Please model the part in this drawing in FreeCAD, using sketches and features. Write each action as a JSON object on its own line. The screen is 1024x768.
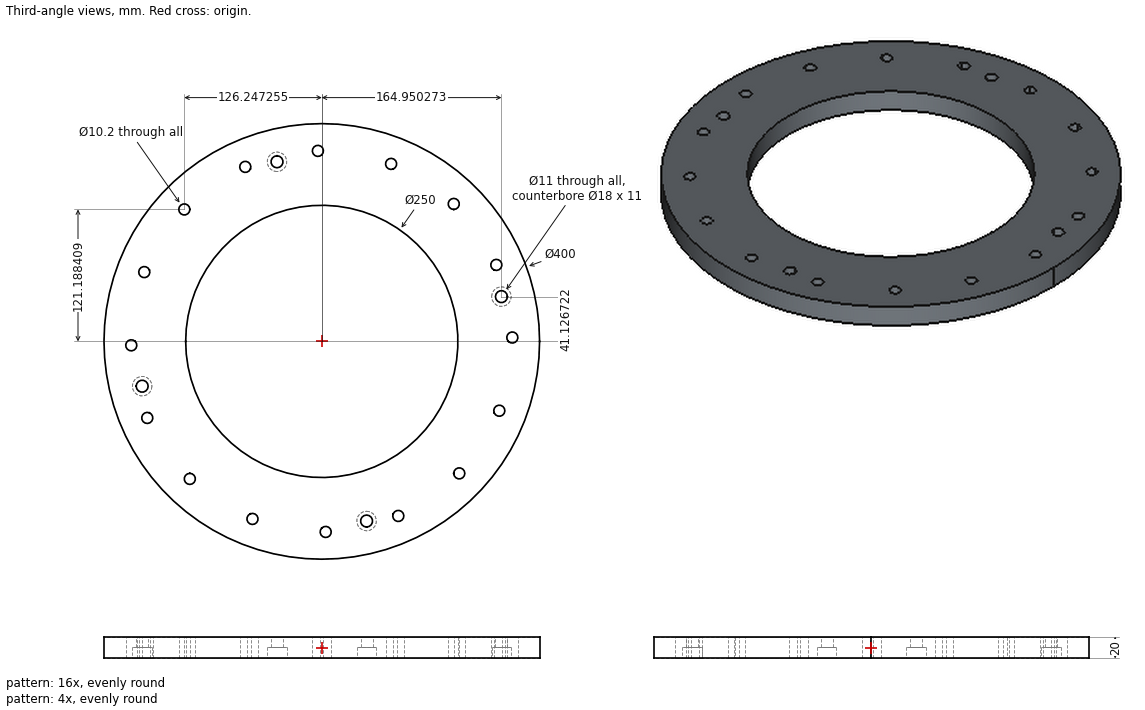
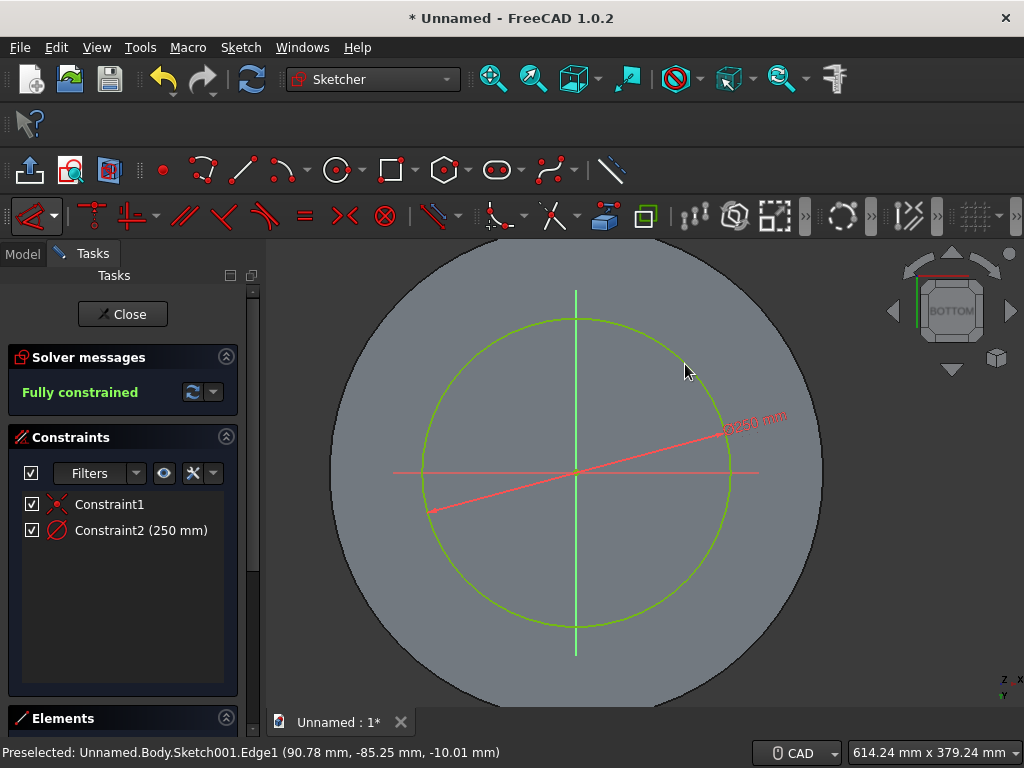
{"action": "left_click", "coordinate": [123, 314]}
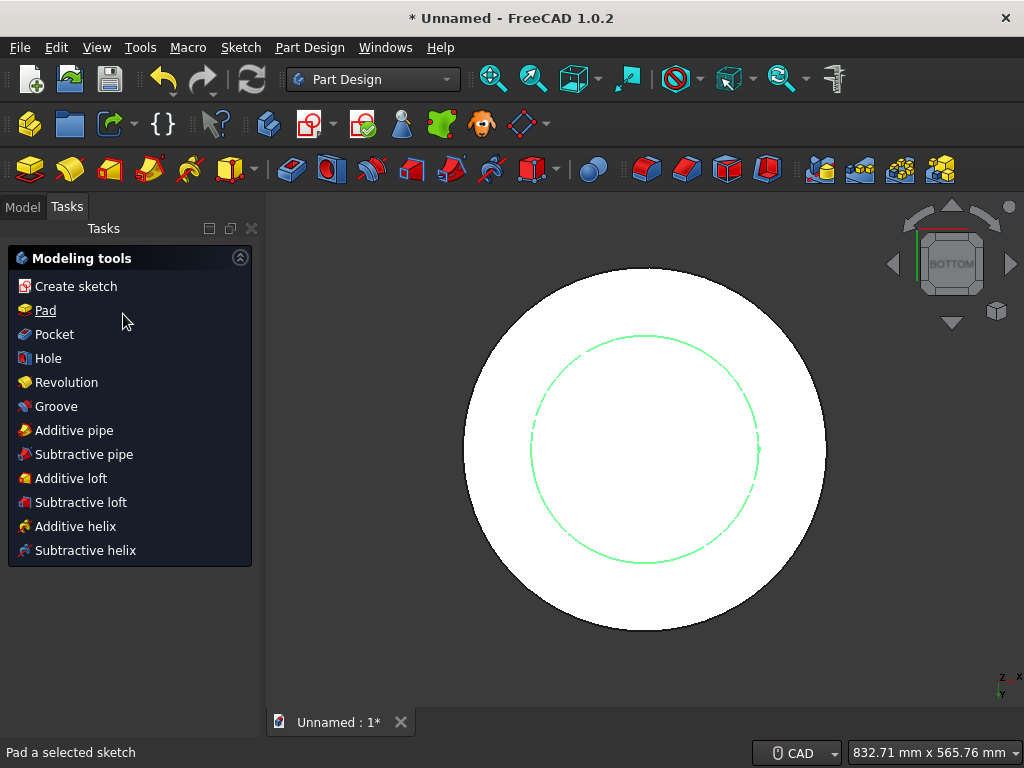
{"action": "left_click", "coordinate": [292, 170]}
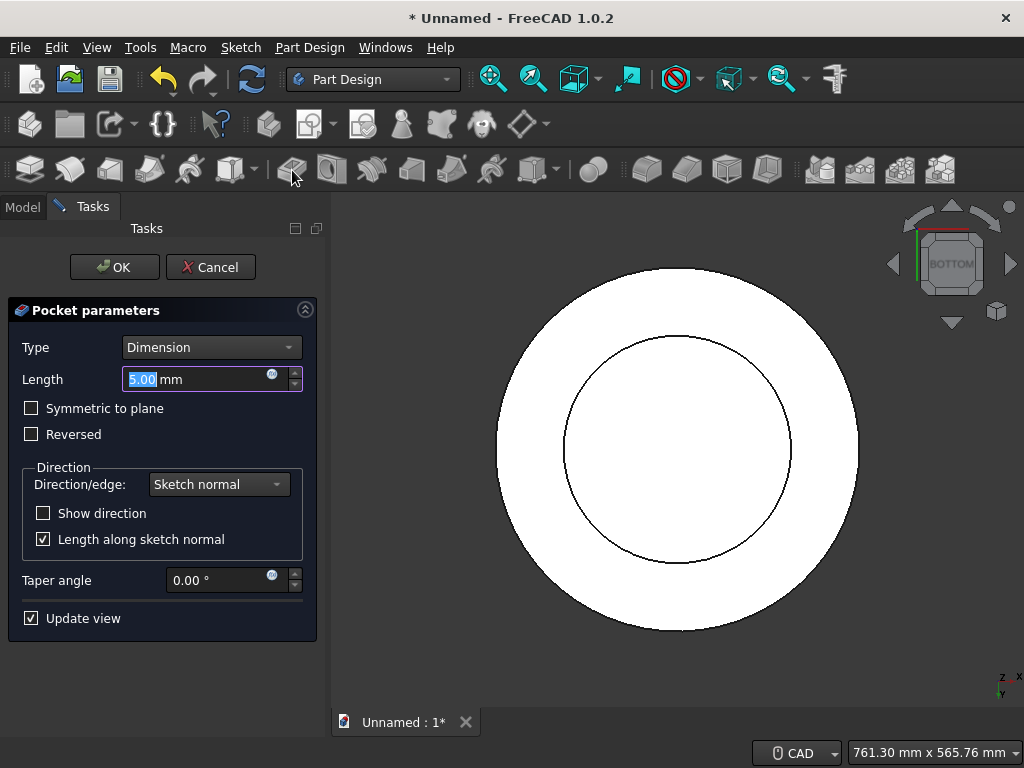
{"action": "left_click", "coordinate": [212, 348]}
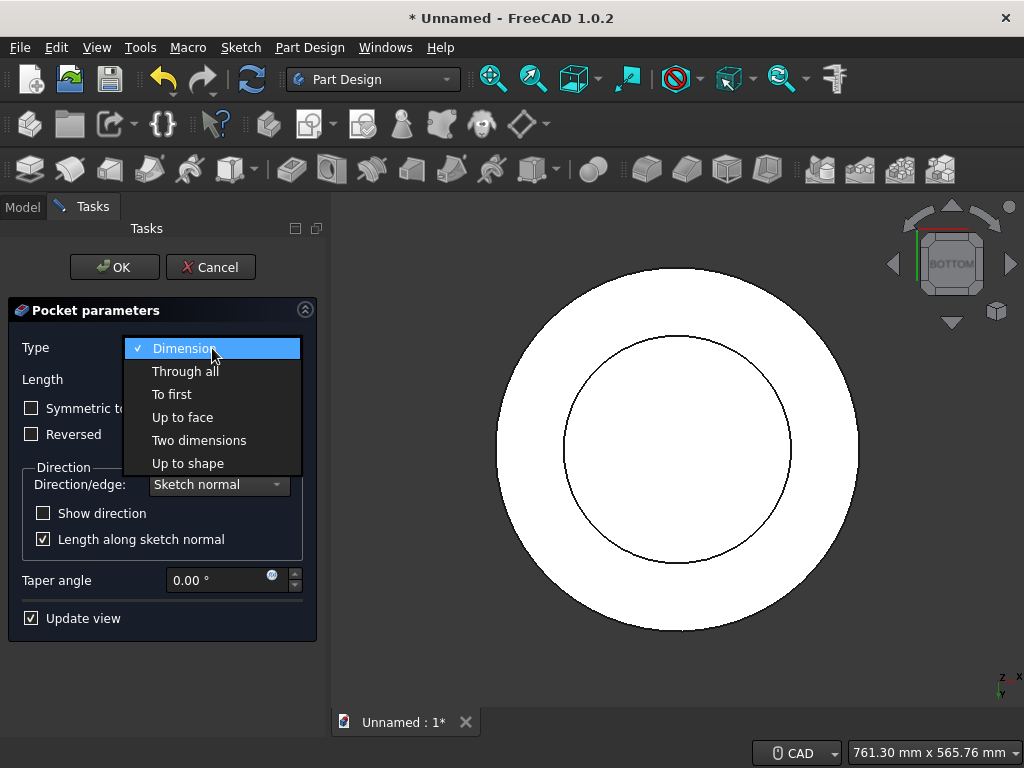
{"action": "left_click", "coordinate": [212, 372]}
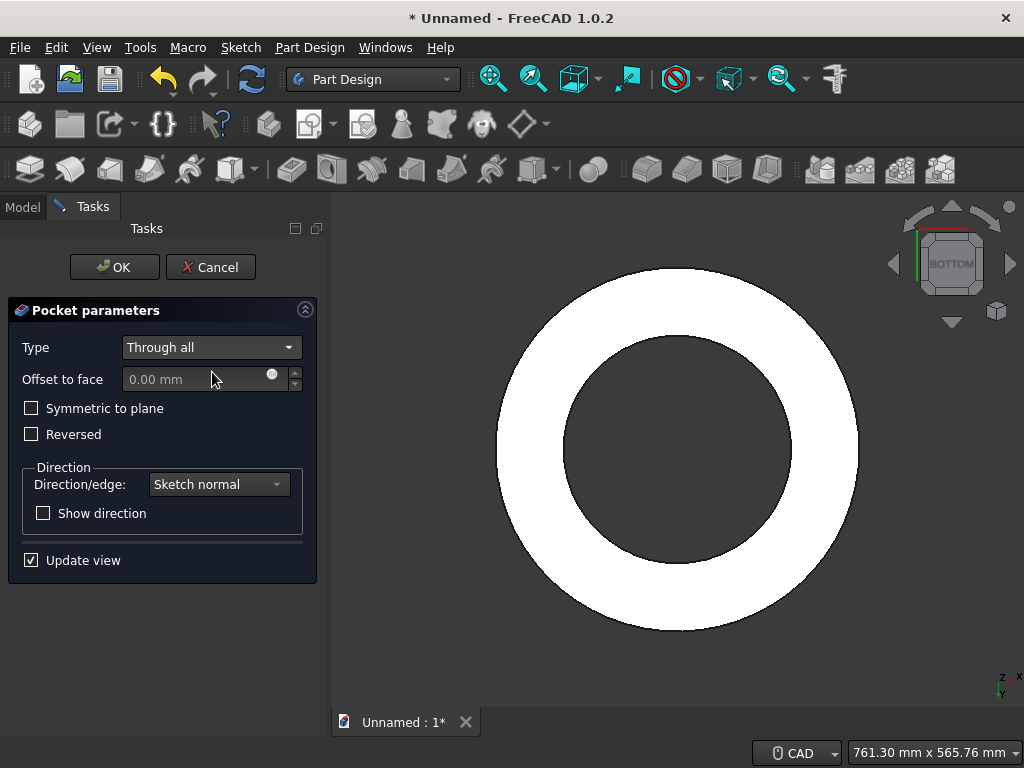
{"action": "left_click", "coordinate": [115, 267]}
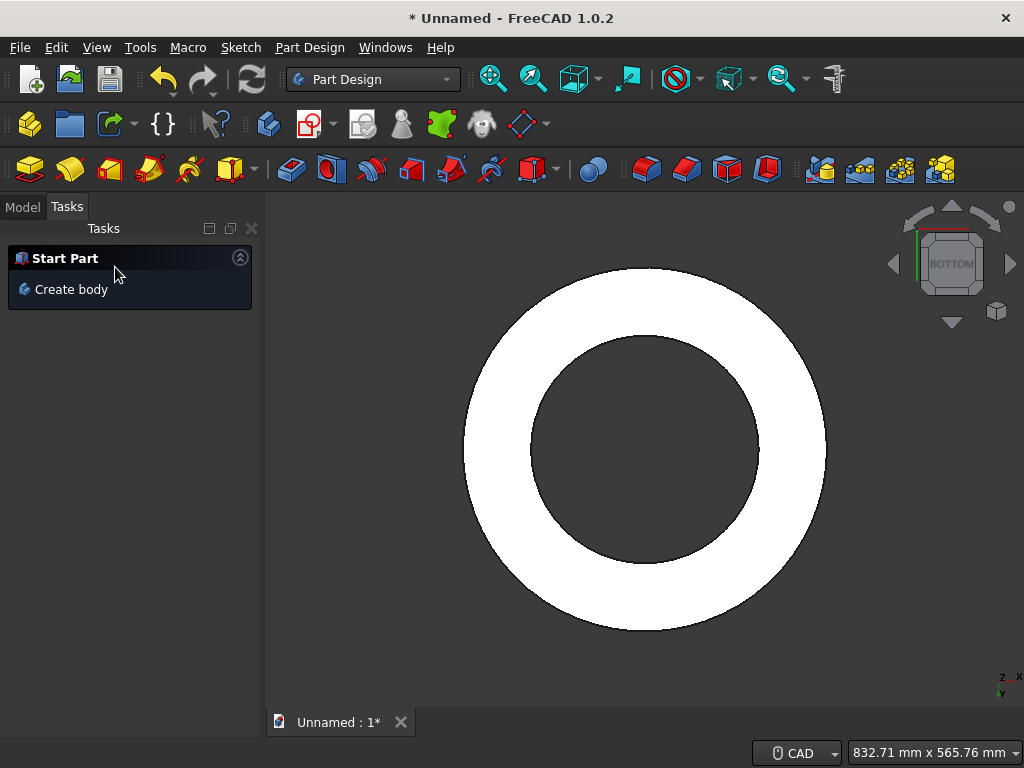
{"action": "left_click", "coordinate": [749, 553]}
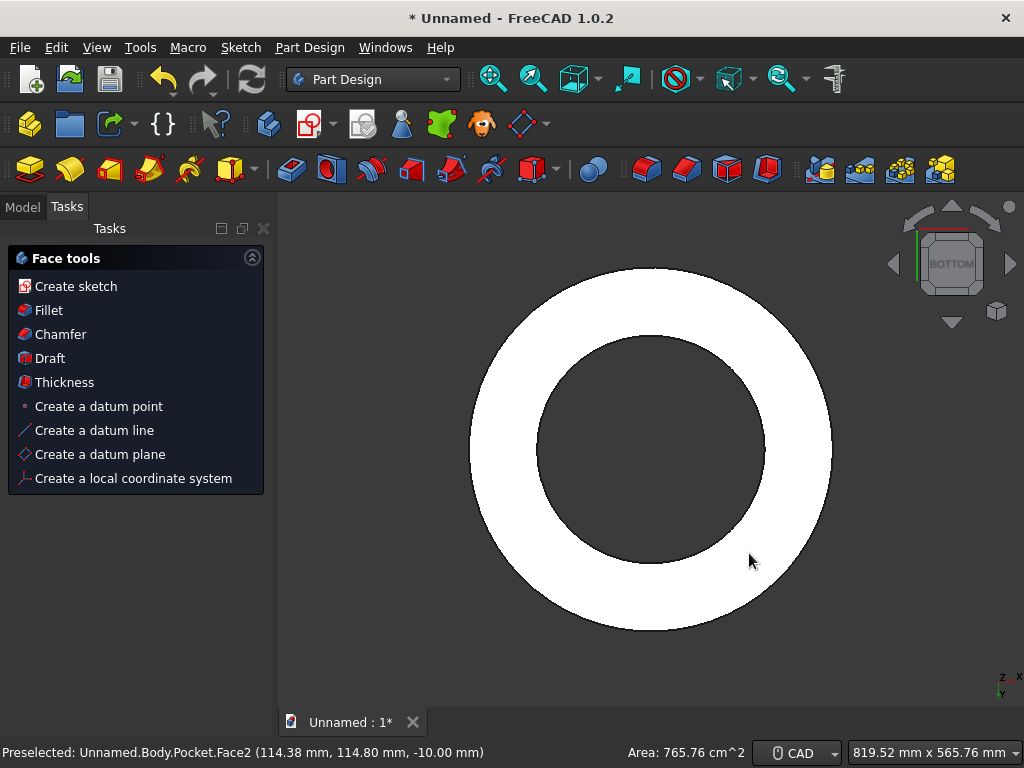
{"action": "left_click", "coordinate": [310, 124]}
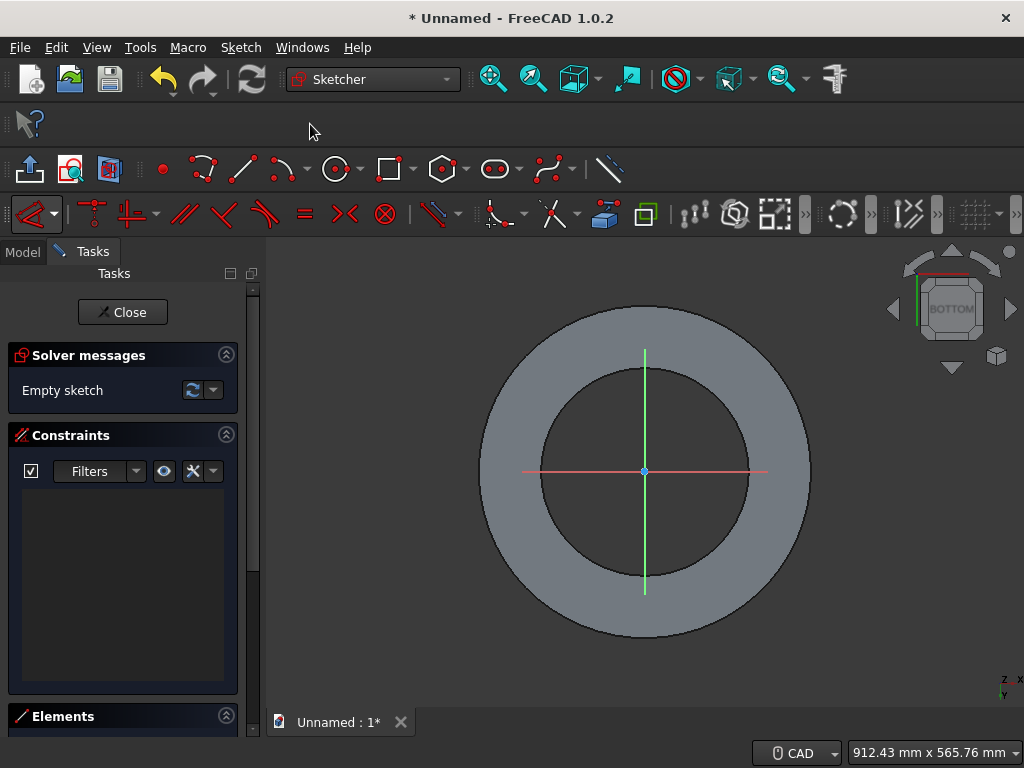
{"action": "scroll", "coordinate": [538, 578], "scroll_direction": "up", "scroll_amount": 15}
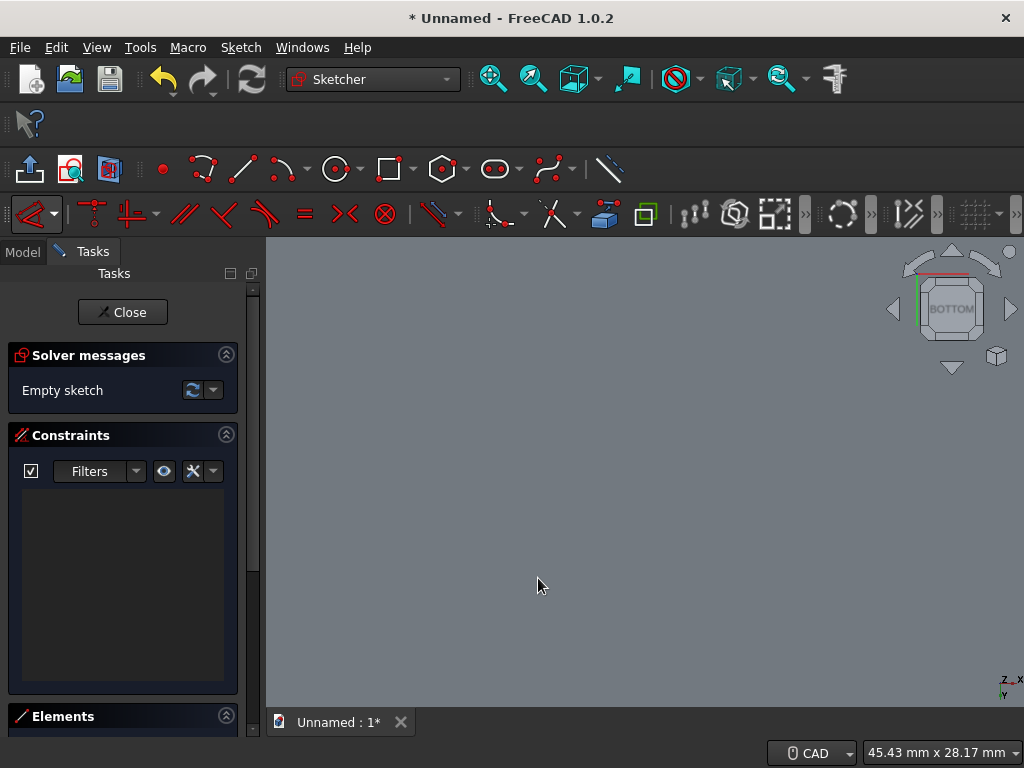
{"action": "scroll", "coordinate": [565, 439], "scroll_direction": "up", "scroll_amount": 3}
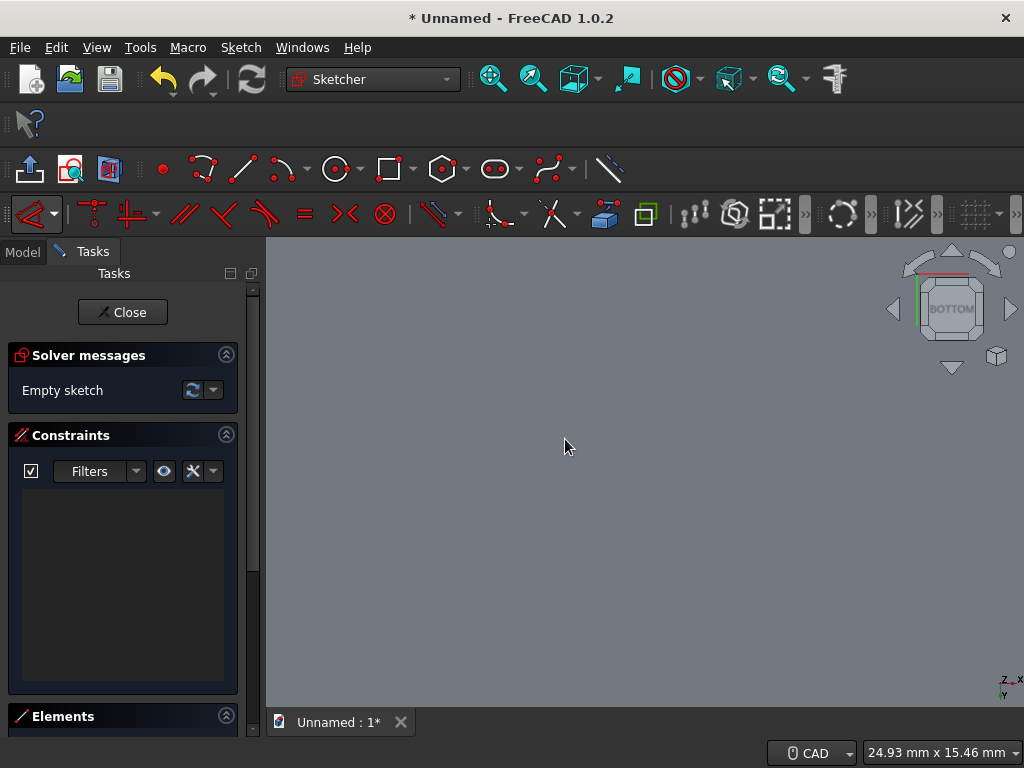
{"action": "left_click", "coordinate": [336, 170]}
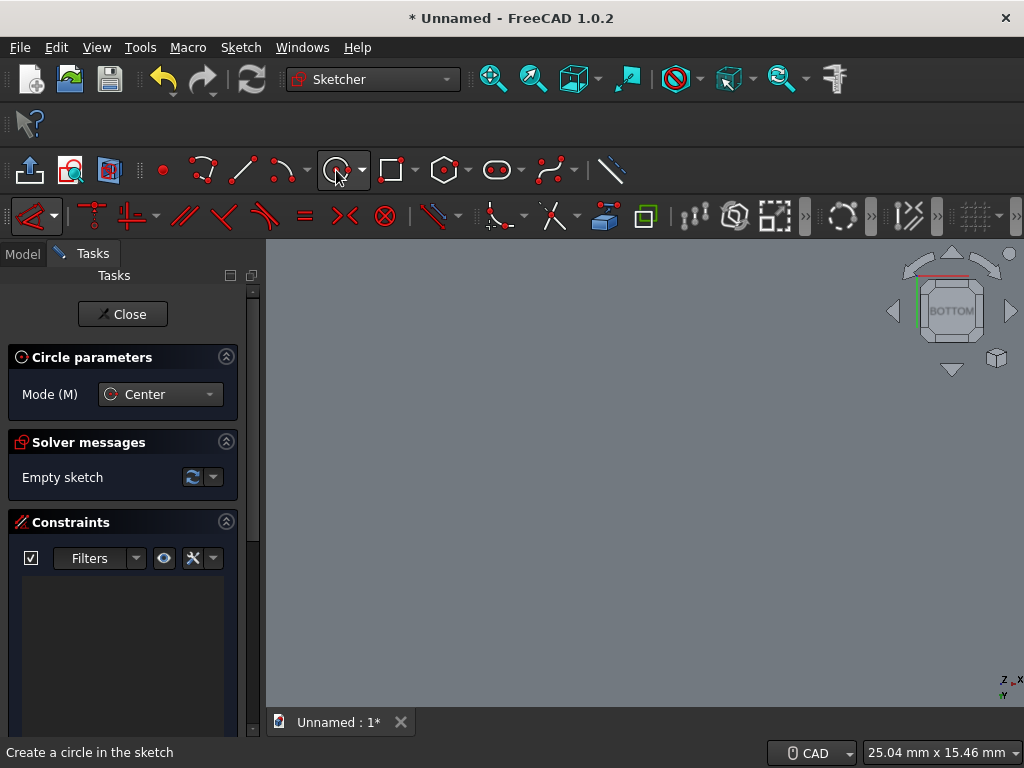
{"action": "left_click", "coordinate": [577, 473]}
{"action": "left_click", "coordinate": [686, 364]}
{"action": "key", "text": "Escape"}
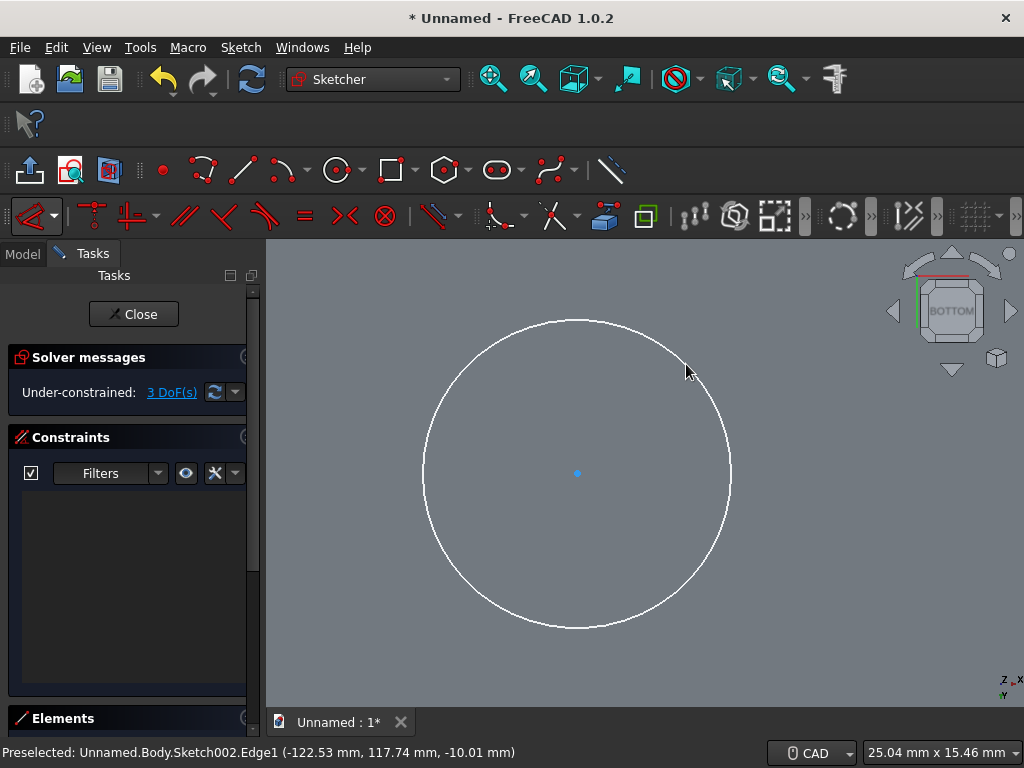
{"action": "left_click", "coordinate": [686, 365]}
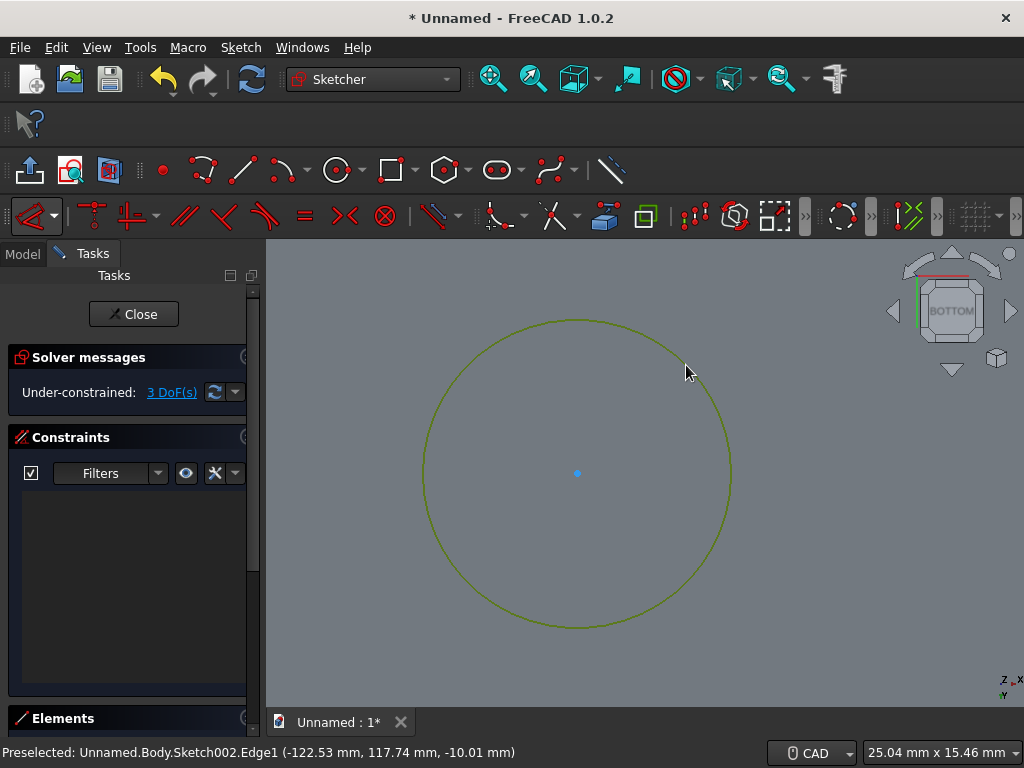
{"action": "left_click", "coordinate": [56, 216]}